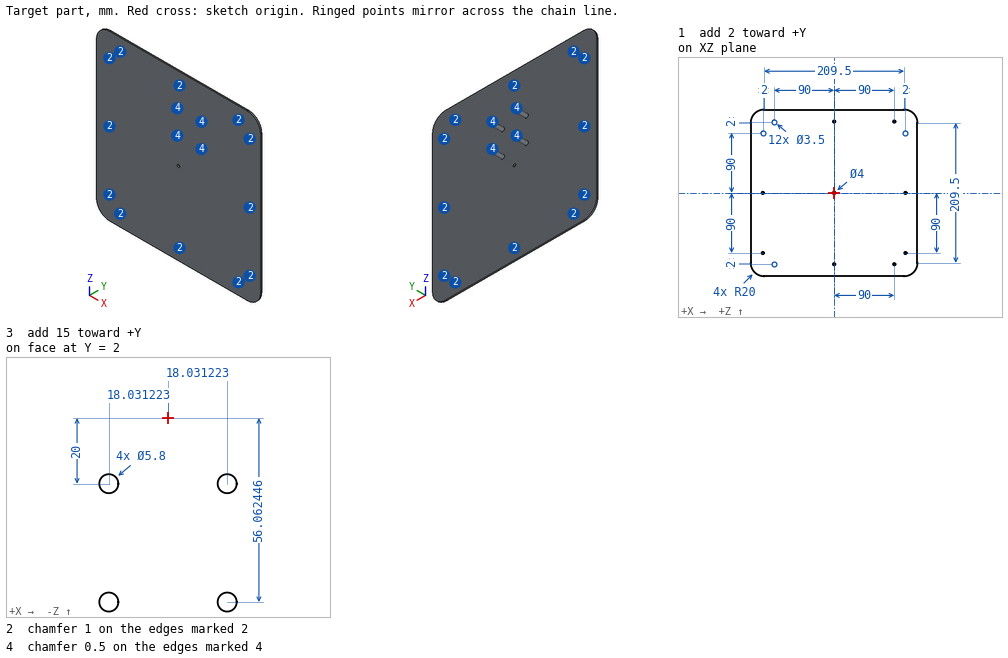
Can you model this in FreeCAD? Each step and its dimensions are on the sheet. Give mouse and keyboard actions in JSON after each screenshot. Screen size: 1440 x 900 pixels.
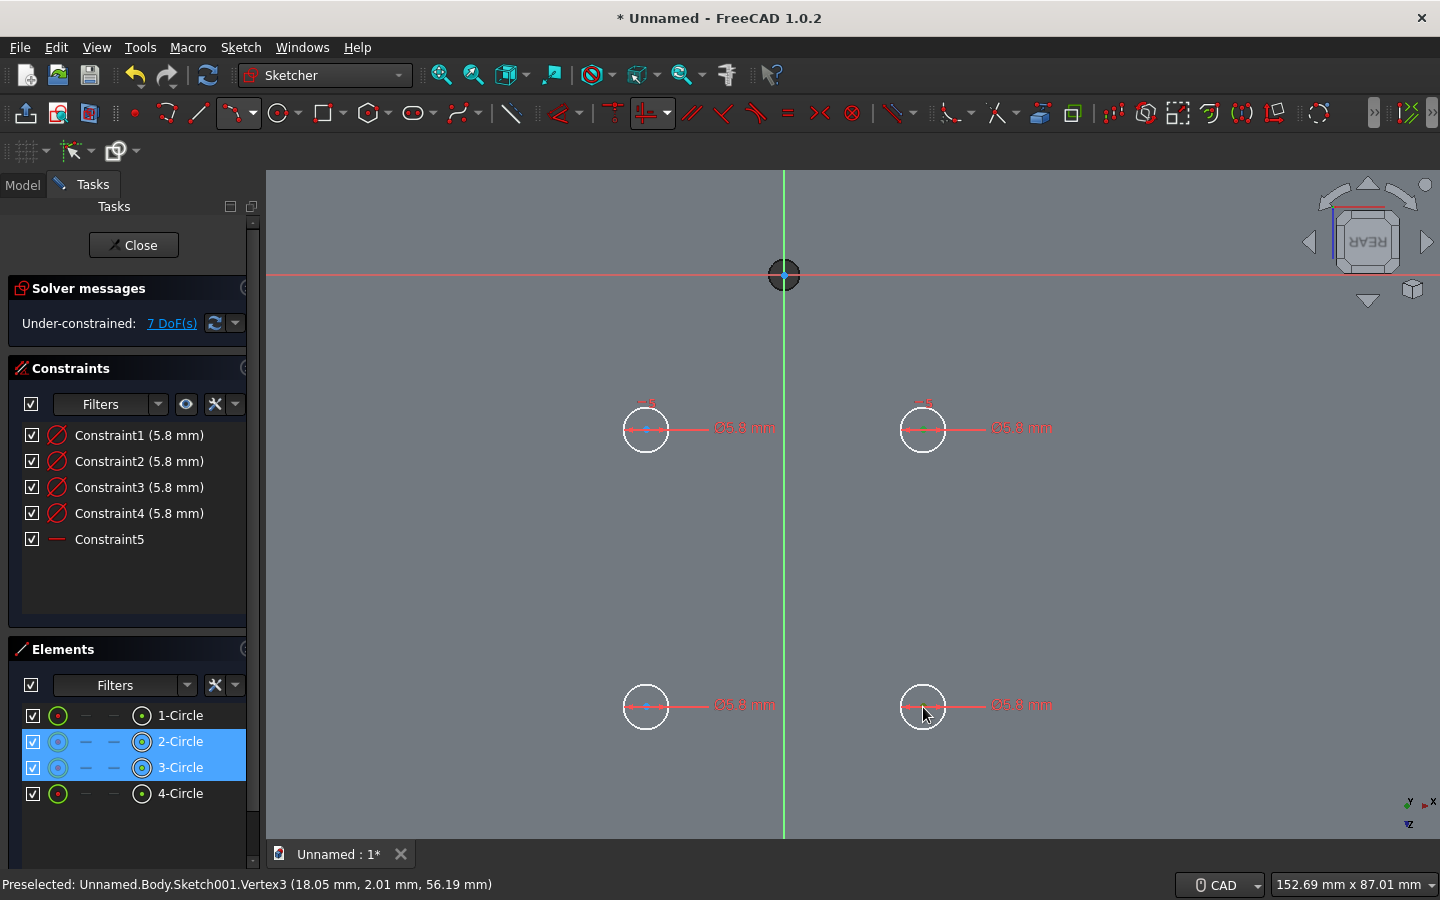
{"action": "key", "text": "v"}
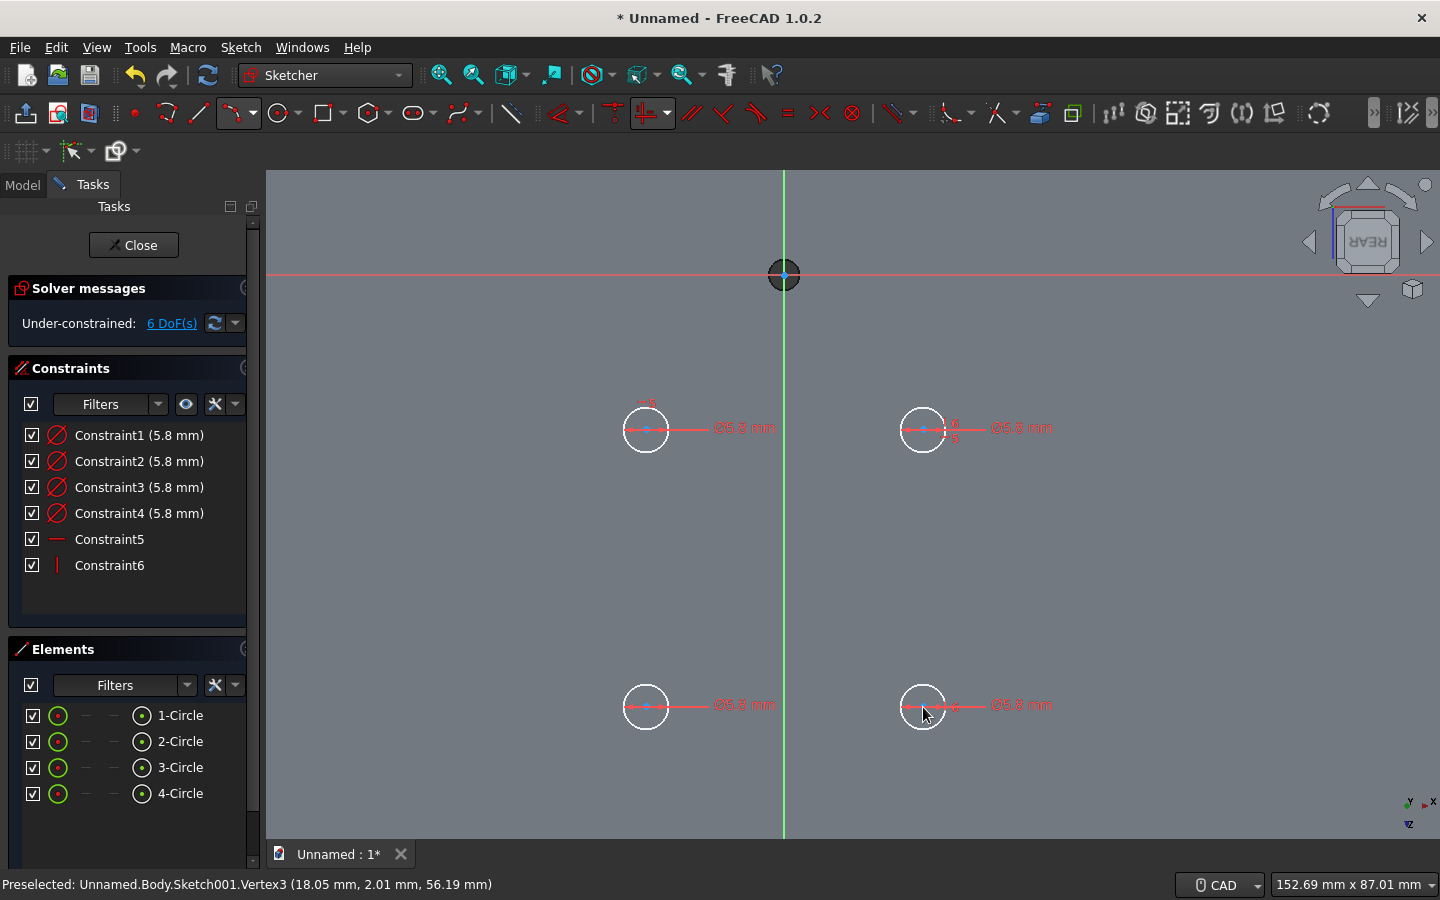
{"action": "left_click", "coordinate": [646, 430]}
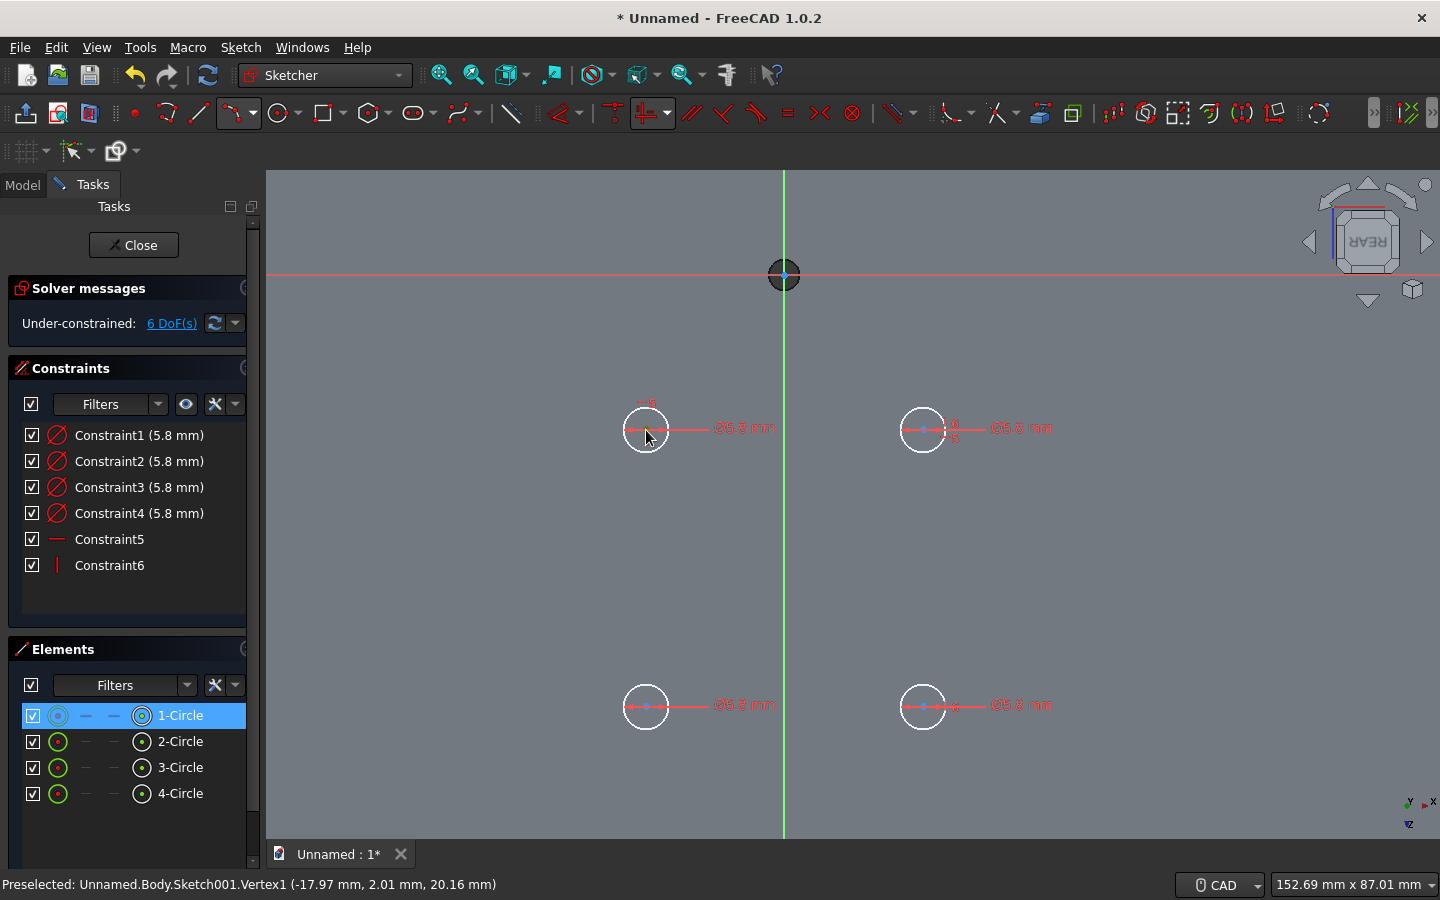
{"action": "left_click", "coordinate": [646, 707]}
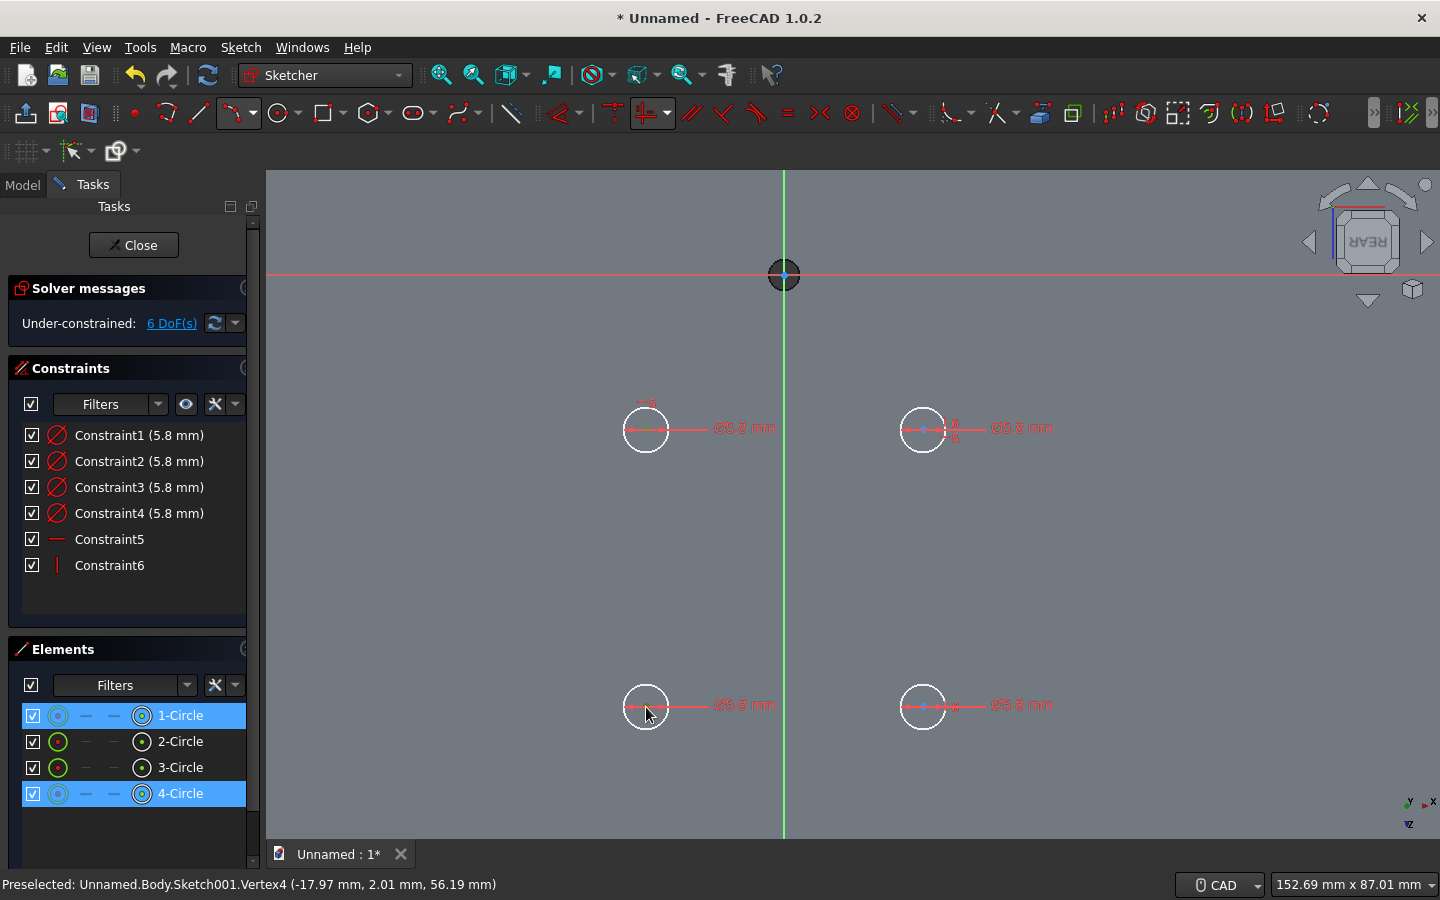
{"action": "left_click", "coordinate": [670, 114]}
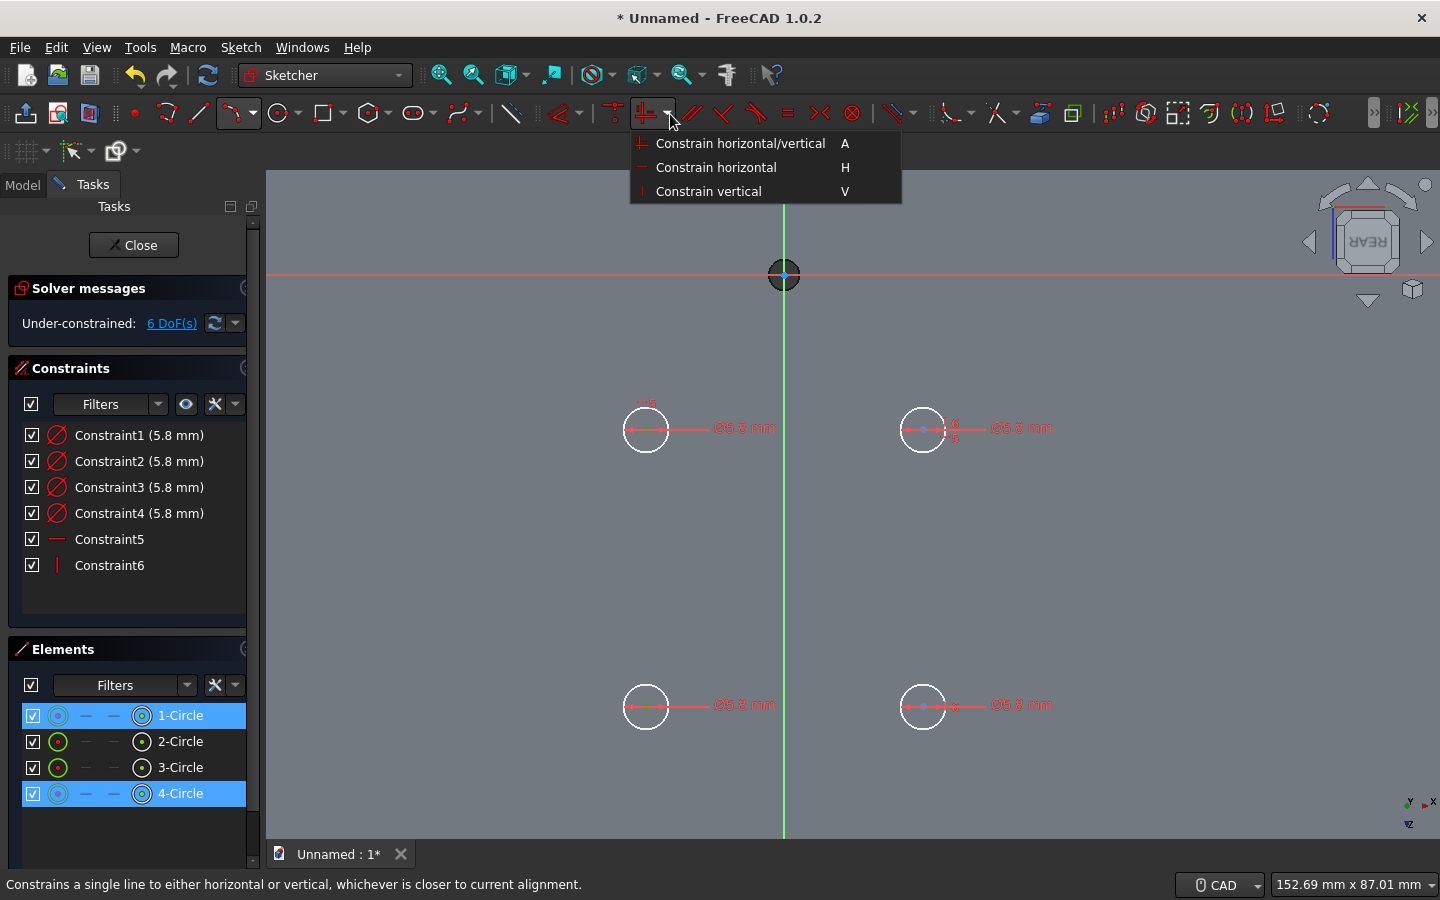
{"action": "left_click", "coordinate": [766, 191]}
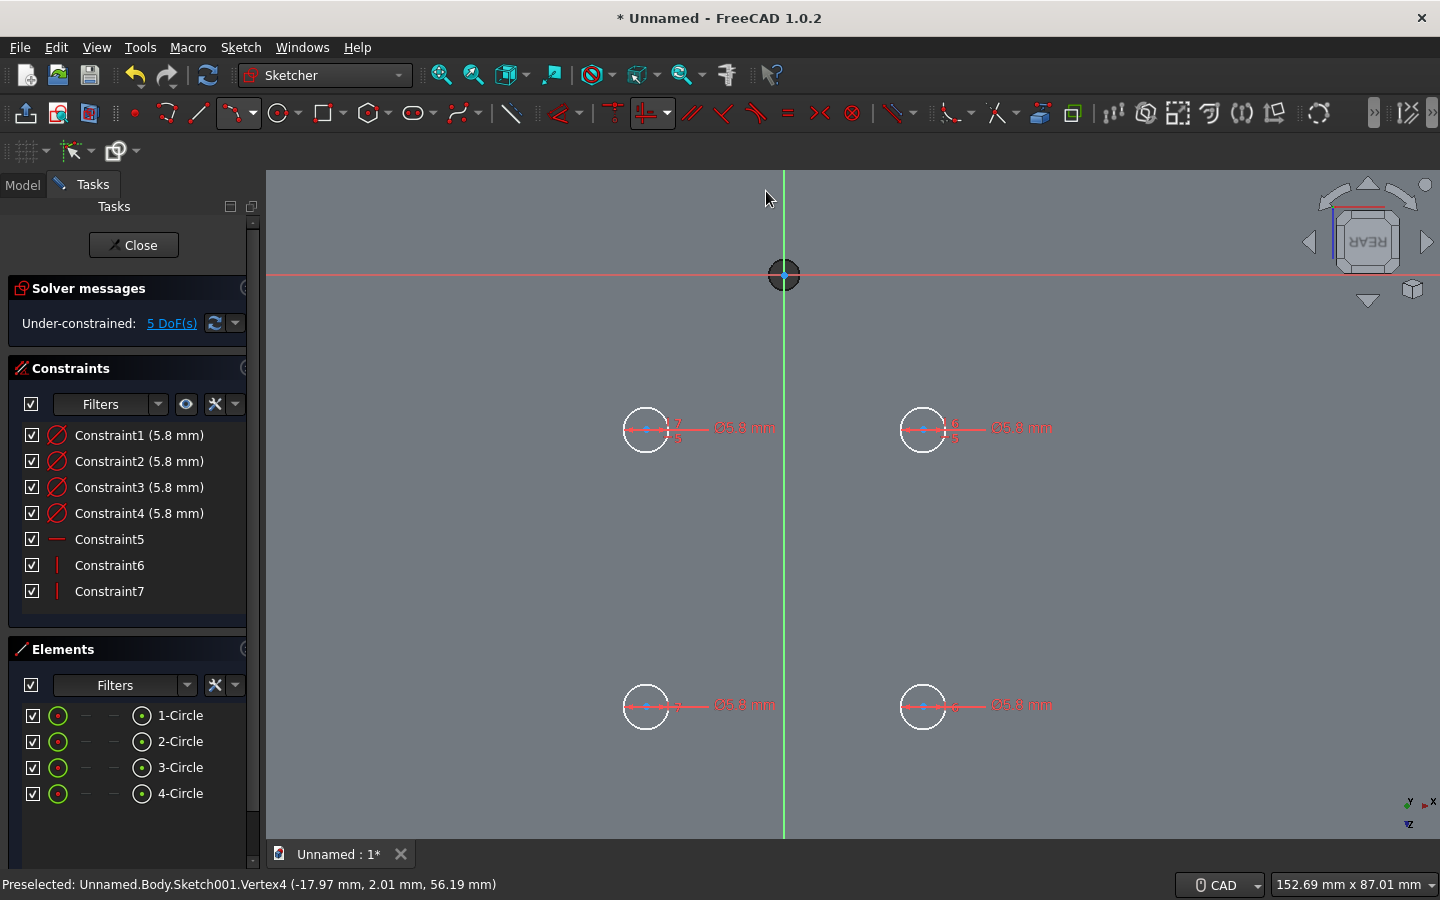
{"action": "left_click", "coordinate": [923, 707]}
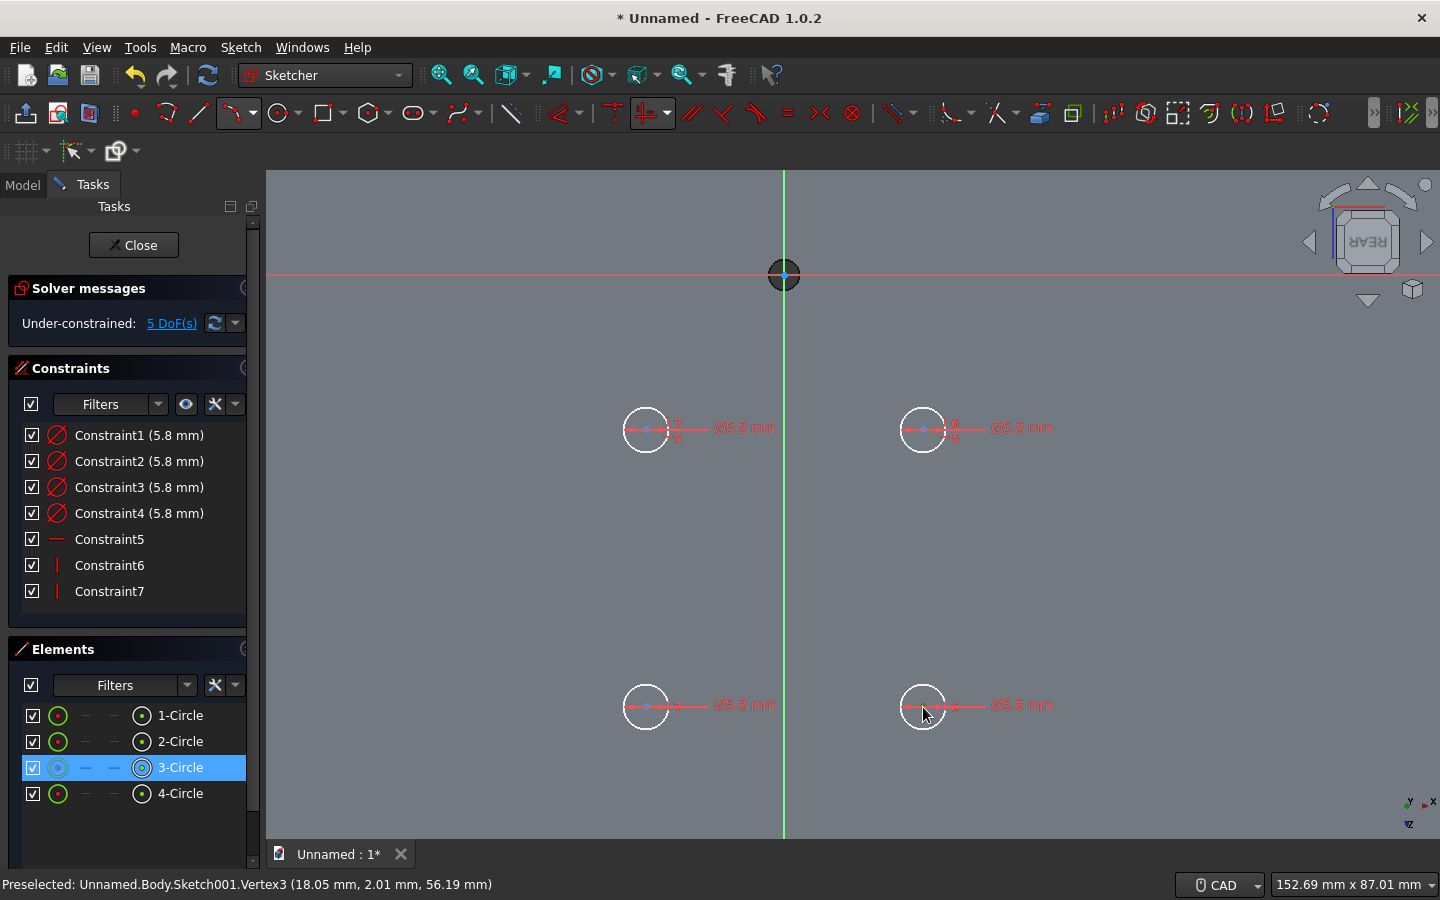
{"action": "left_click", "coordinate": [646, 707]}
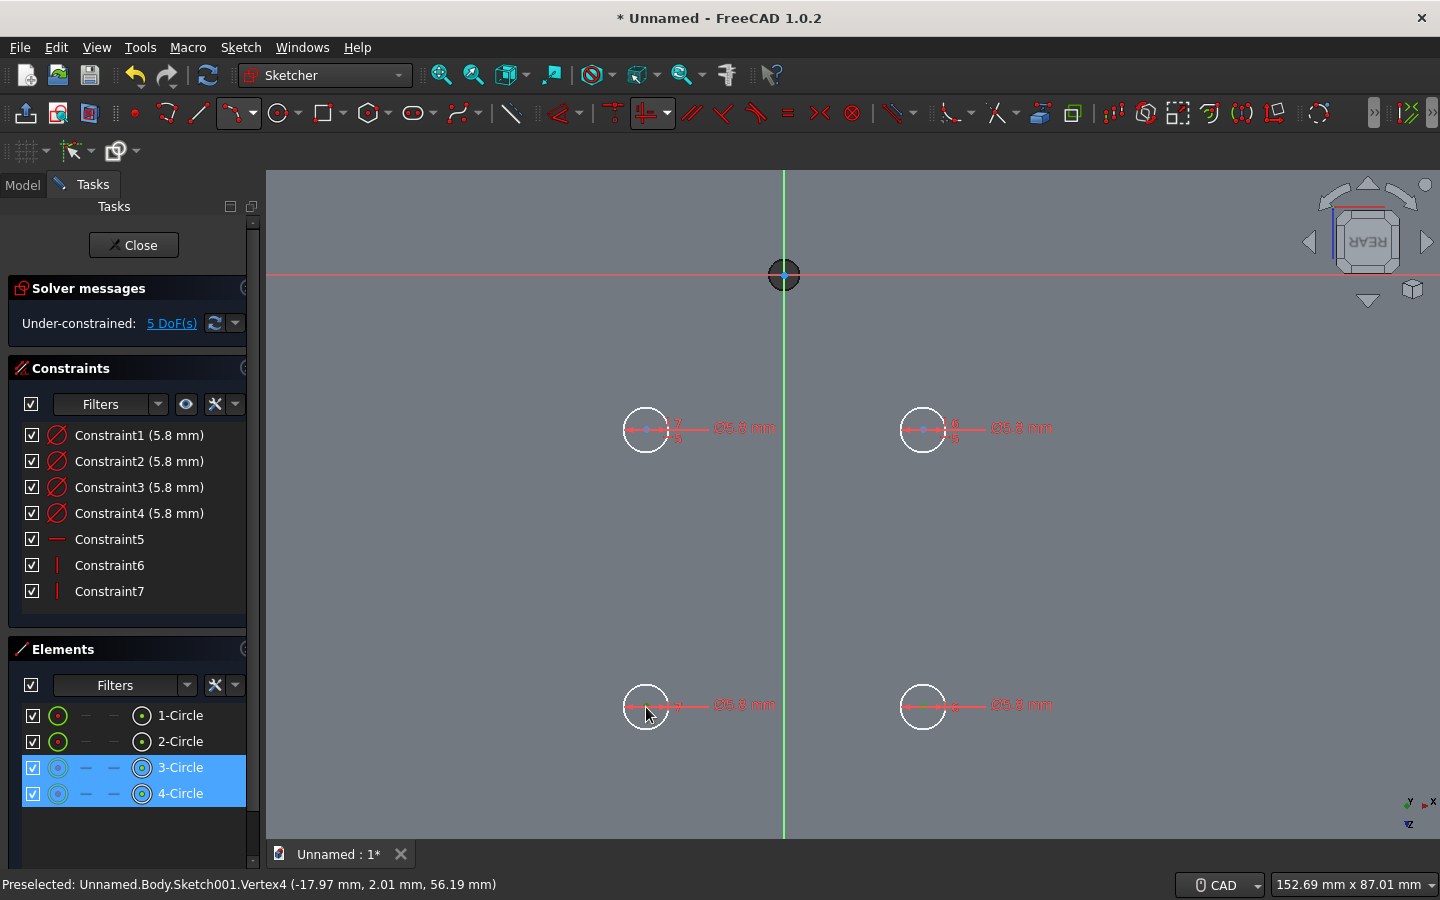
{"action": "key", "text": "h"}